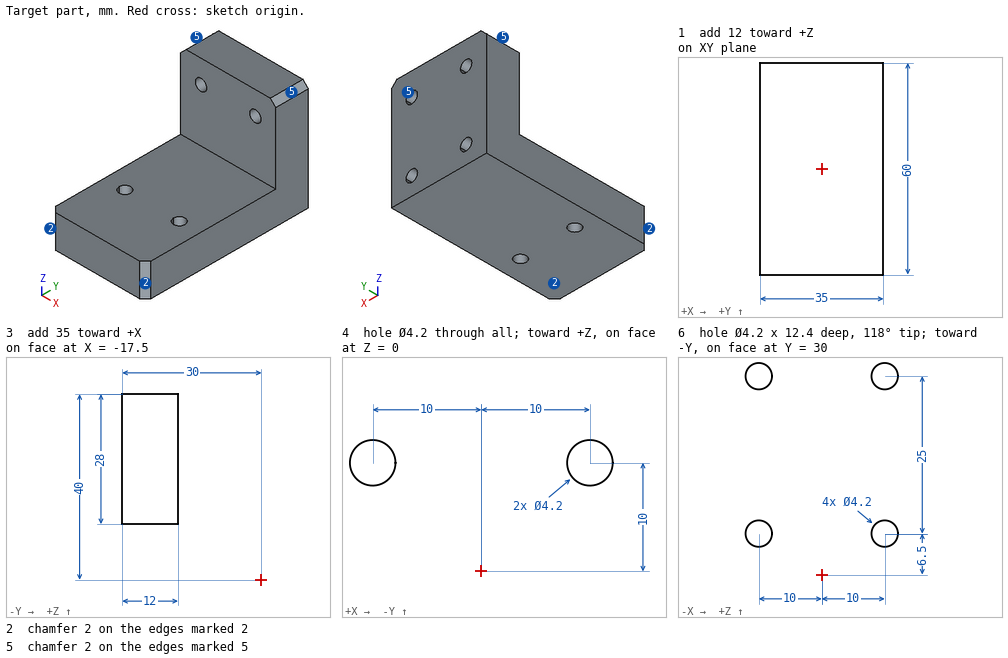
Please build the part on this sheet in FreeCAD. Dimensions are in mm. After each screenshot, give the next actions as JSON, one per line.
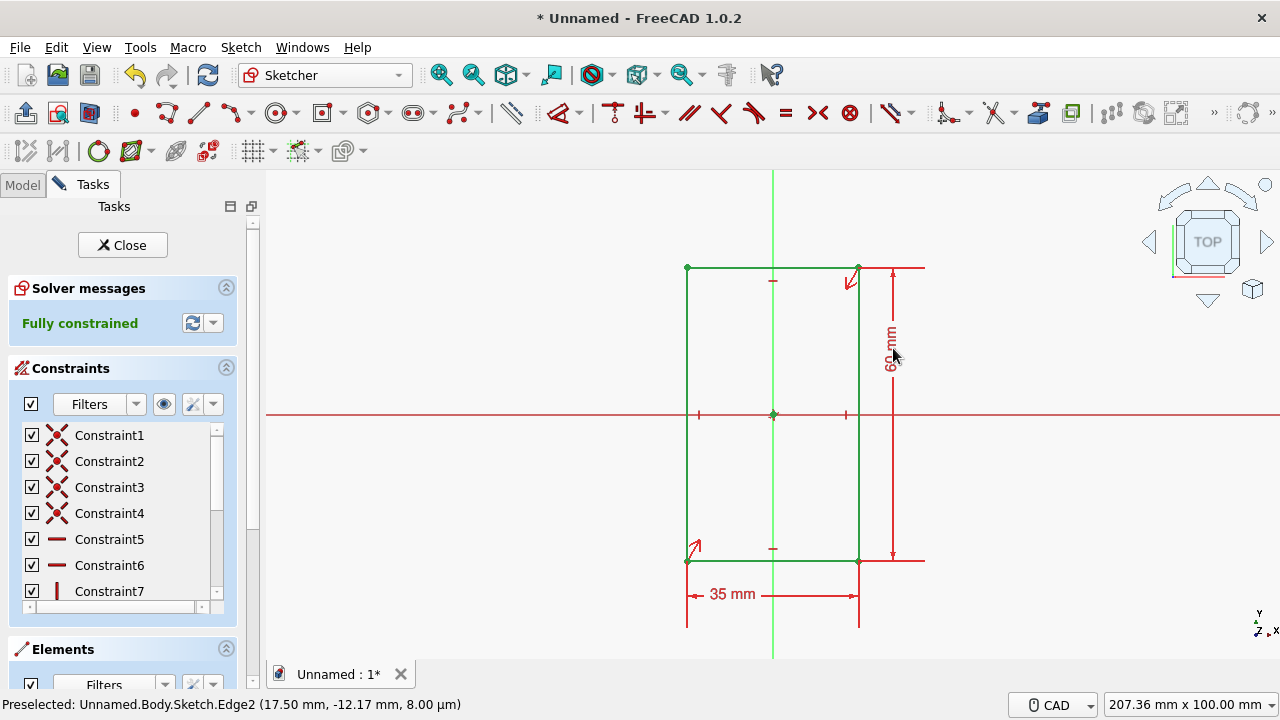
{"action": "left_click", "coordinate": [123, 245]}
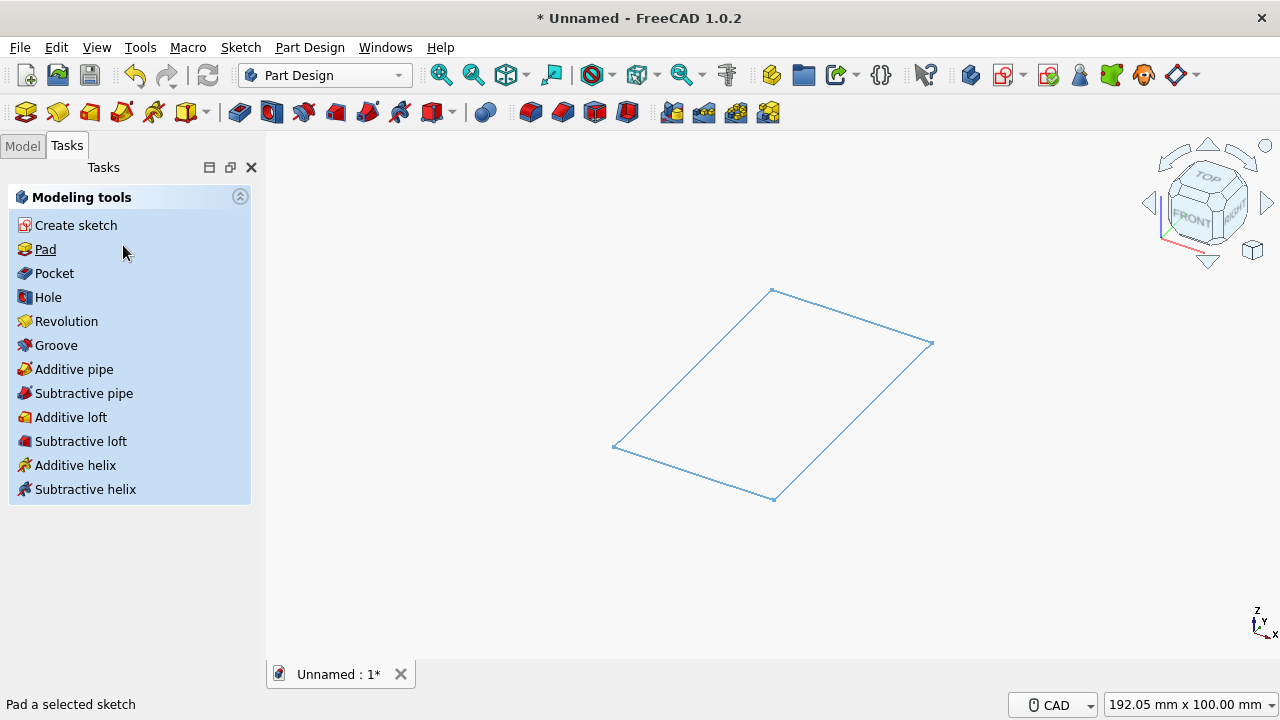
{"action": "left_click", "coordinate": [26, 112]}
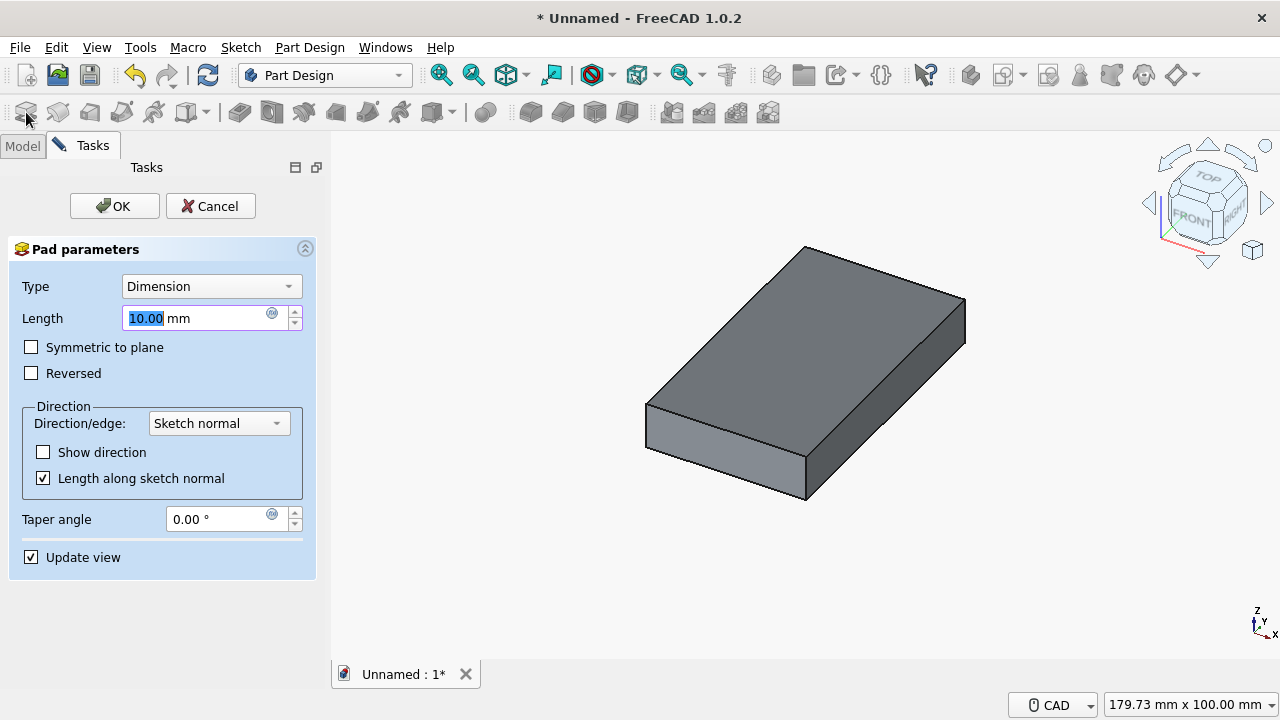
{"action": "type", "text": "12"}
{"action": "key", "text": "Tab"}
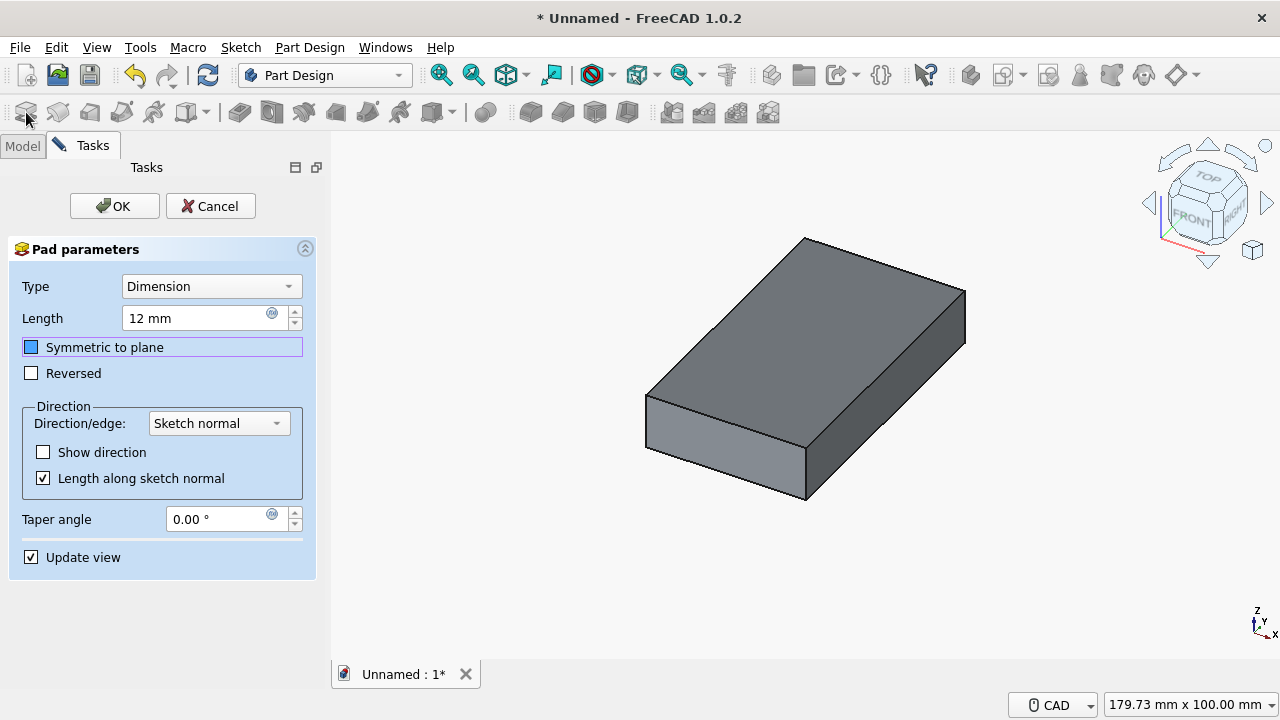
{"action": "left_click", "coordinate": [115, 206]}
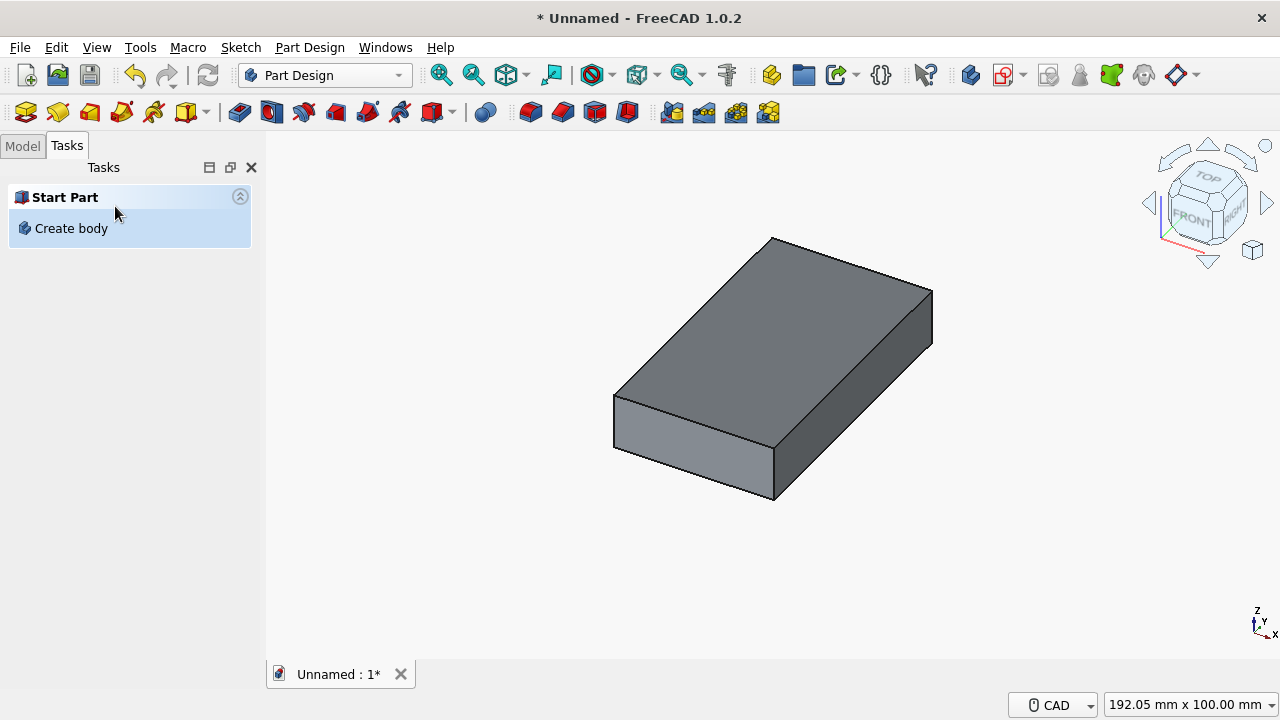
{"action": "left_click", "coordinate": [774, 473]}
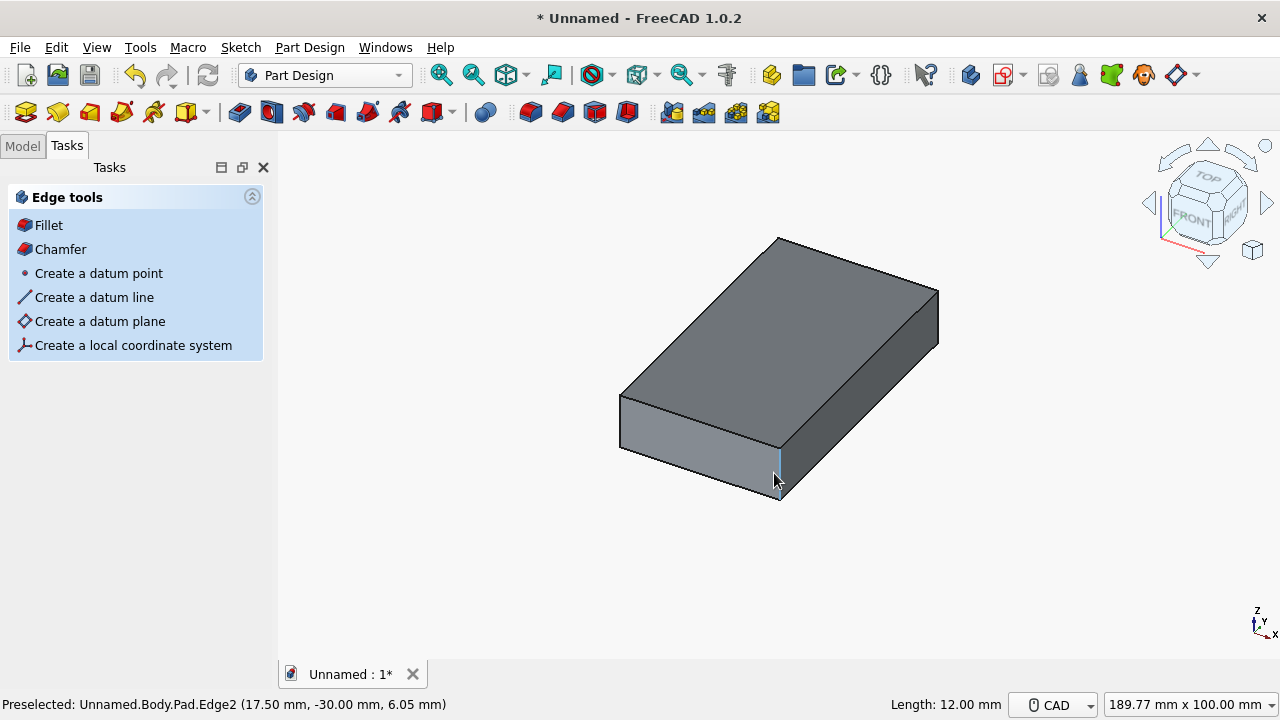
{"action": "key", "text": "0"}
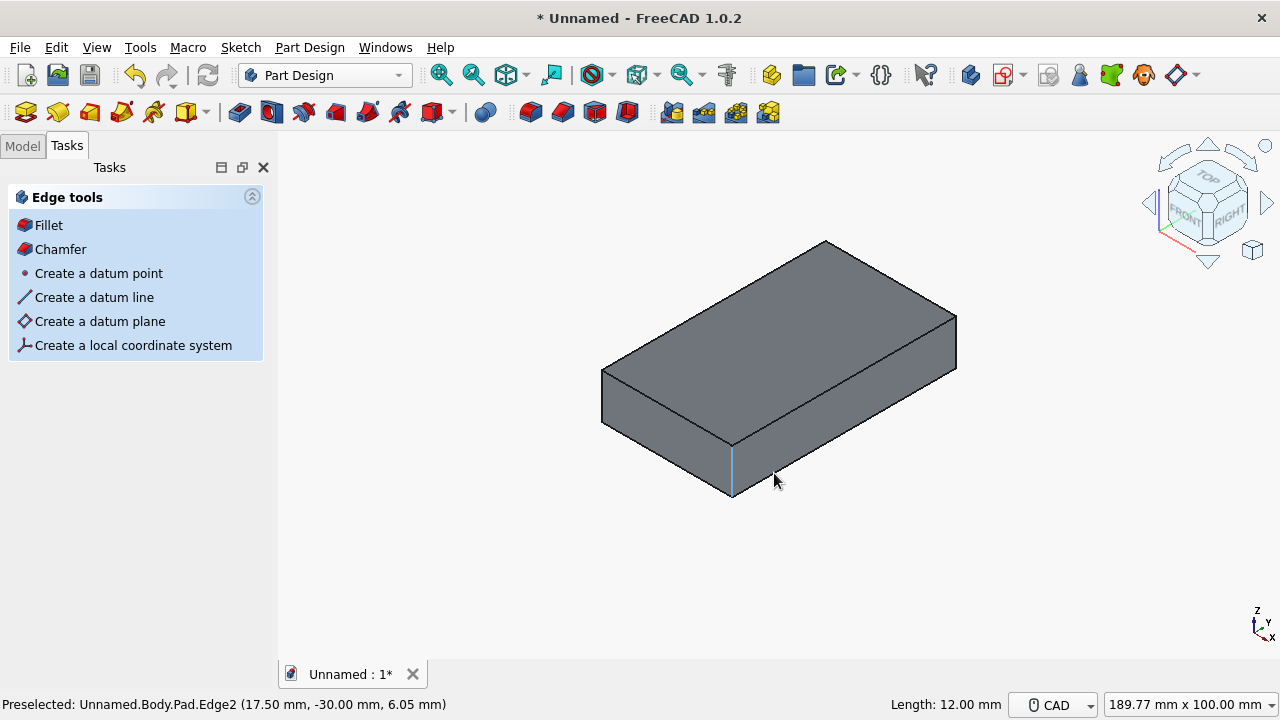
{"action": "key", "text": "2"}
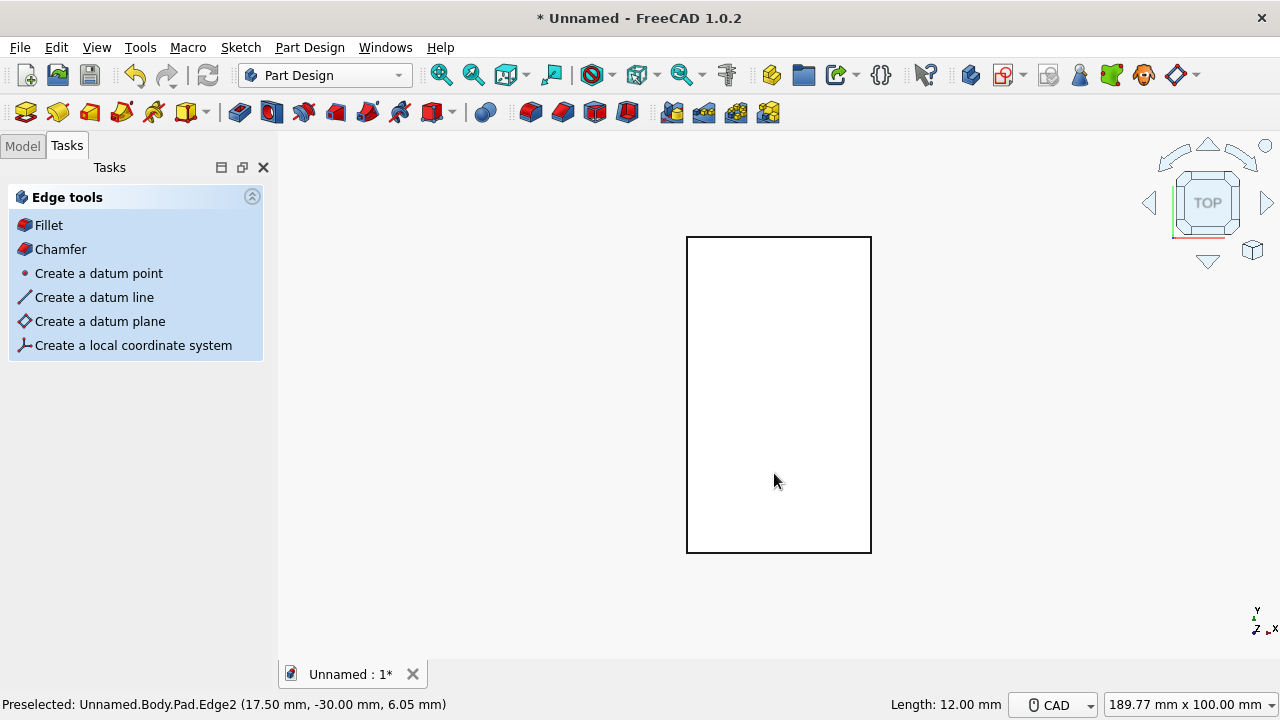
{"action": "key", "text": "1"}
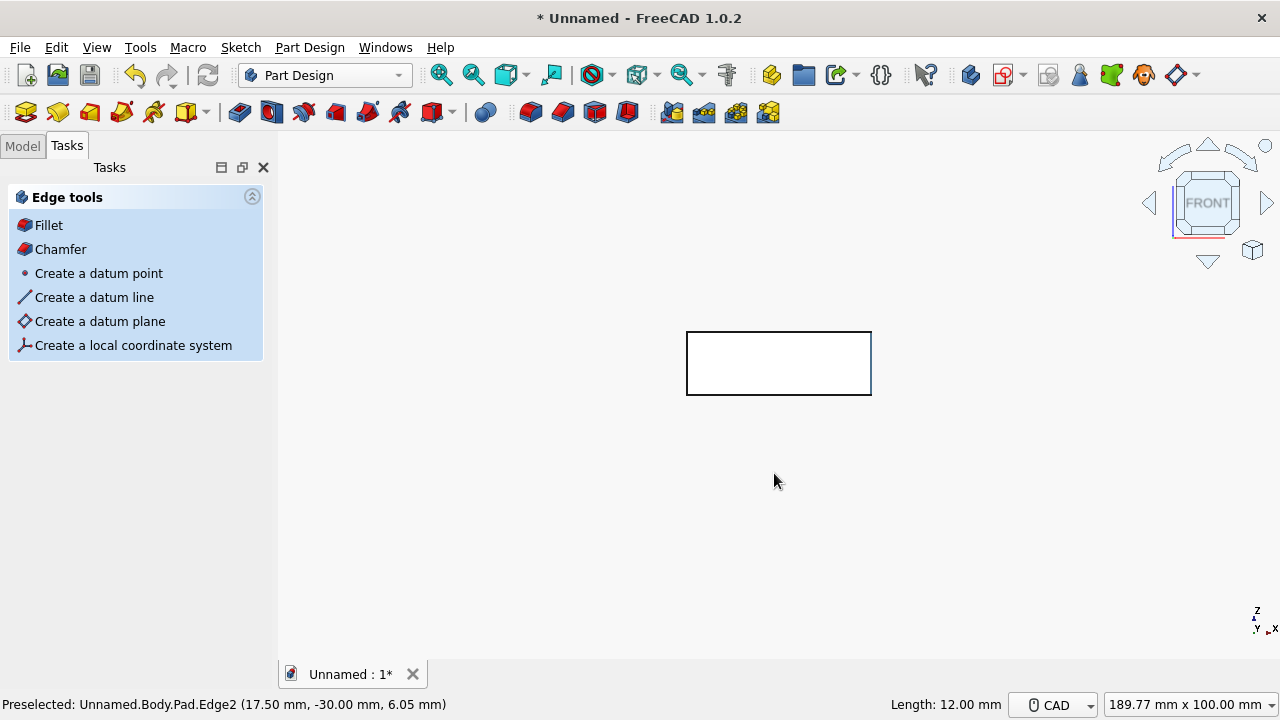
{"action": "left_click", "coordinate": [442, 76]}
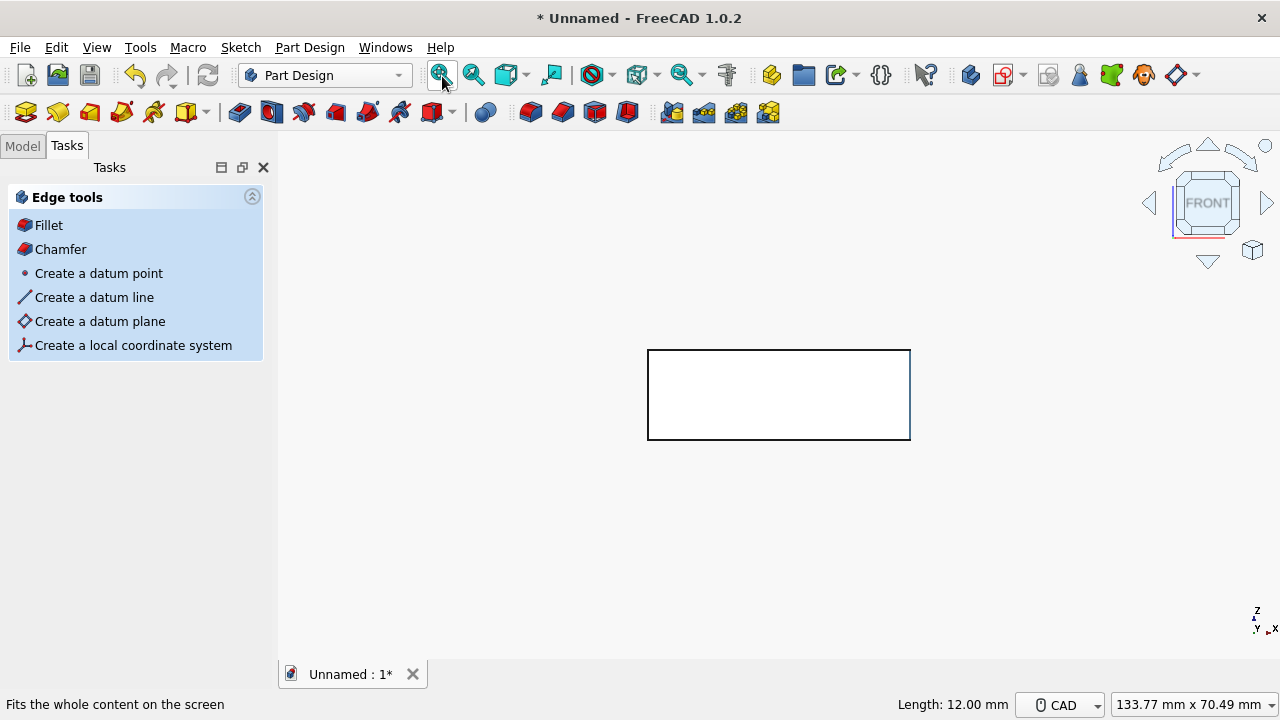
{"action": "left_click", "coordinate": [648, 394], "text": "ctrl"}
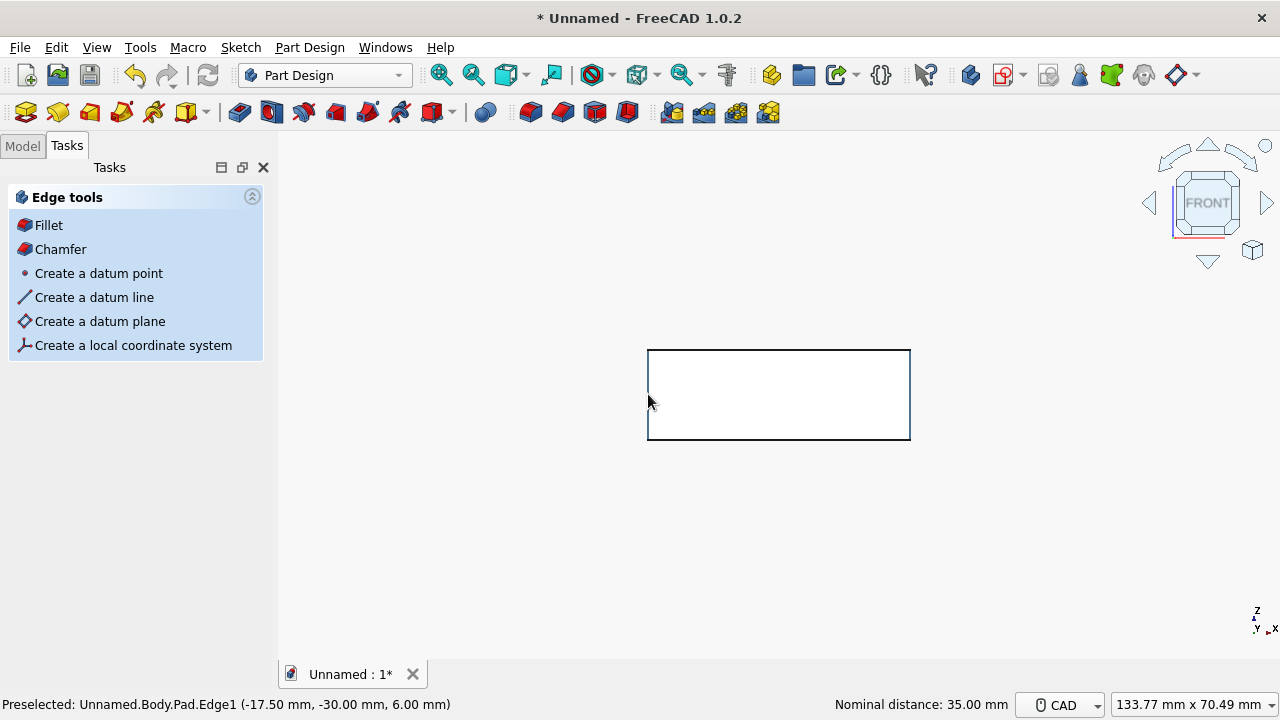
{"action": "left_click", "coordinate": [564, 112]}